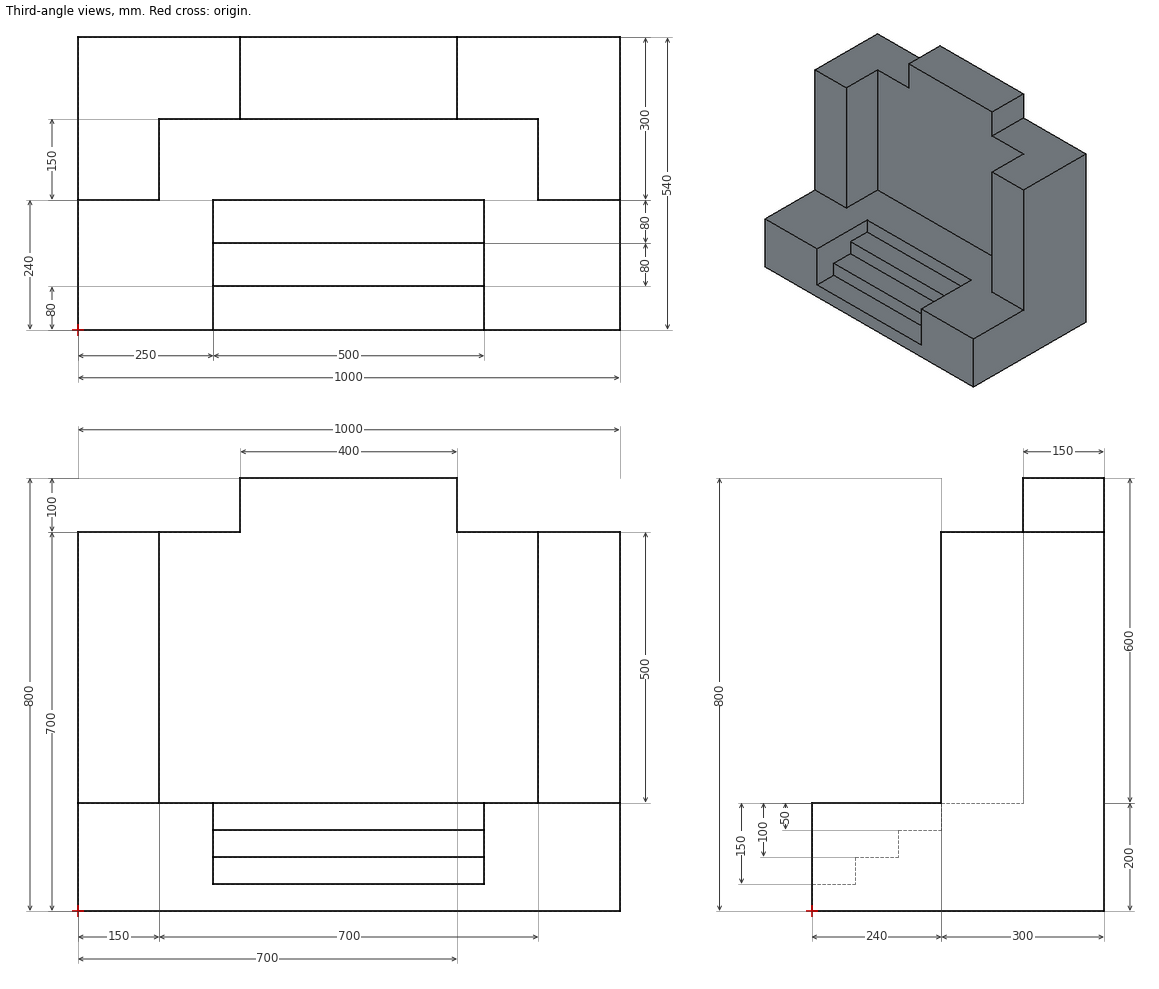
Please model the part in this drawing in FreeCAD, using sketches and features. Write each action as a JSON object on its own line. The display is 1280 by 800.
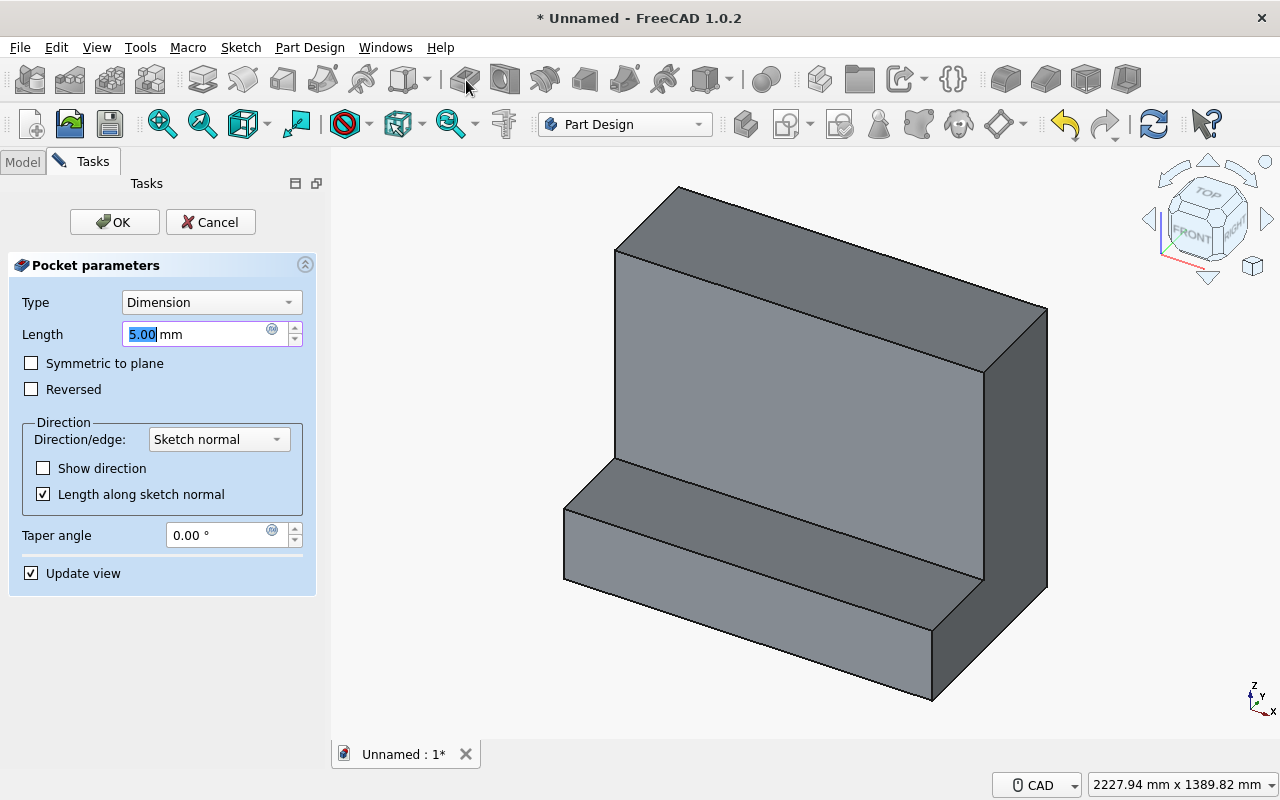
{"action": "type", "text": "100"}
{"action": "key", "text": "Tab"}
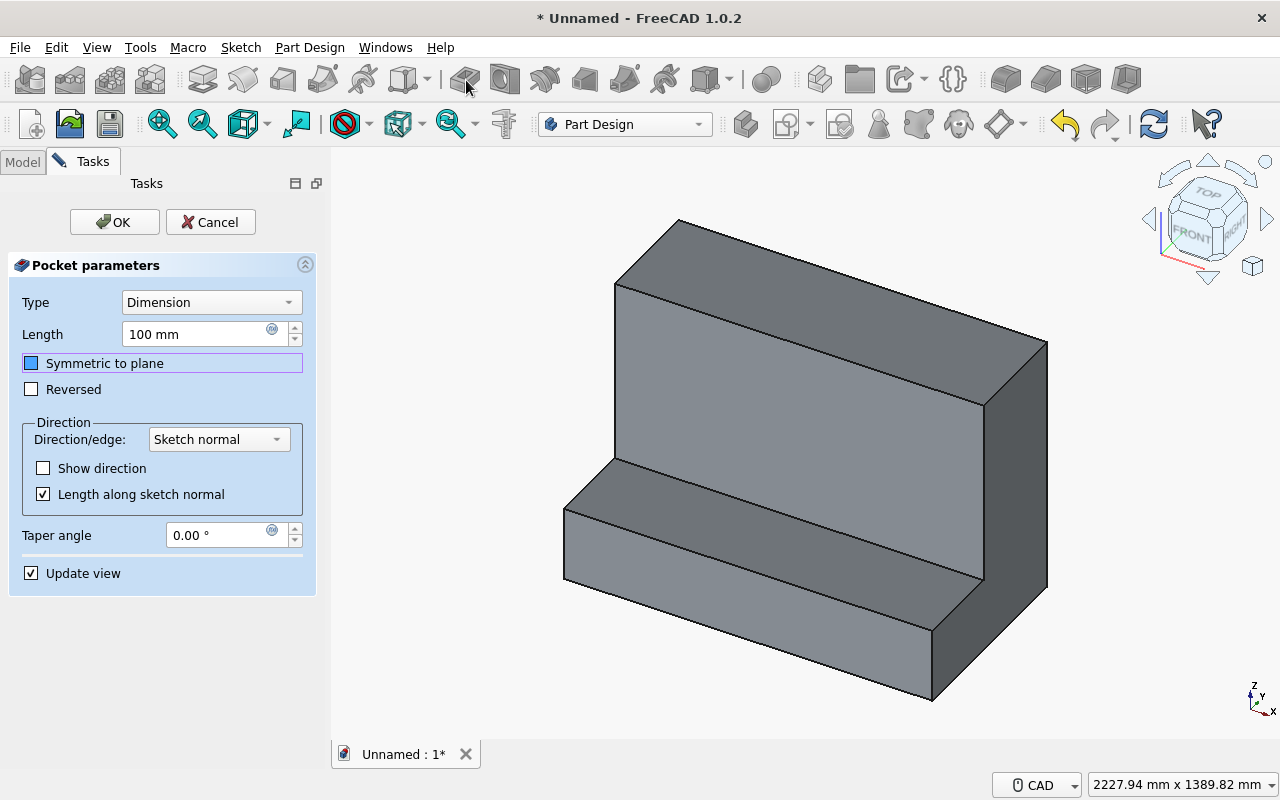
{"action": "left_click", "coordinate": [115, 222]}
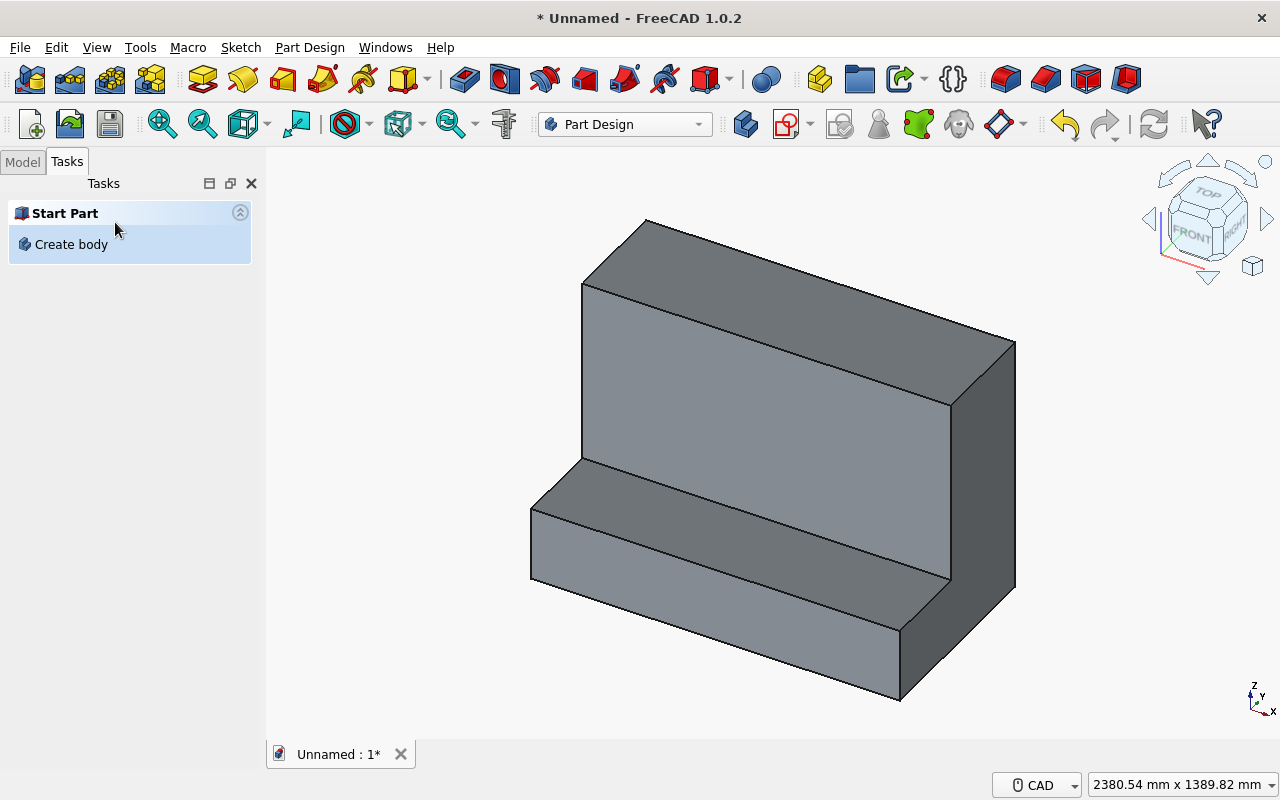
{"action": "key", "text": "4"}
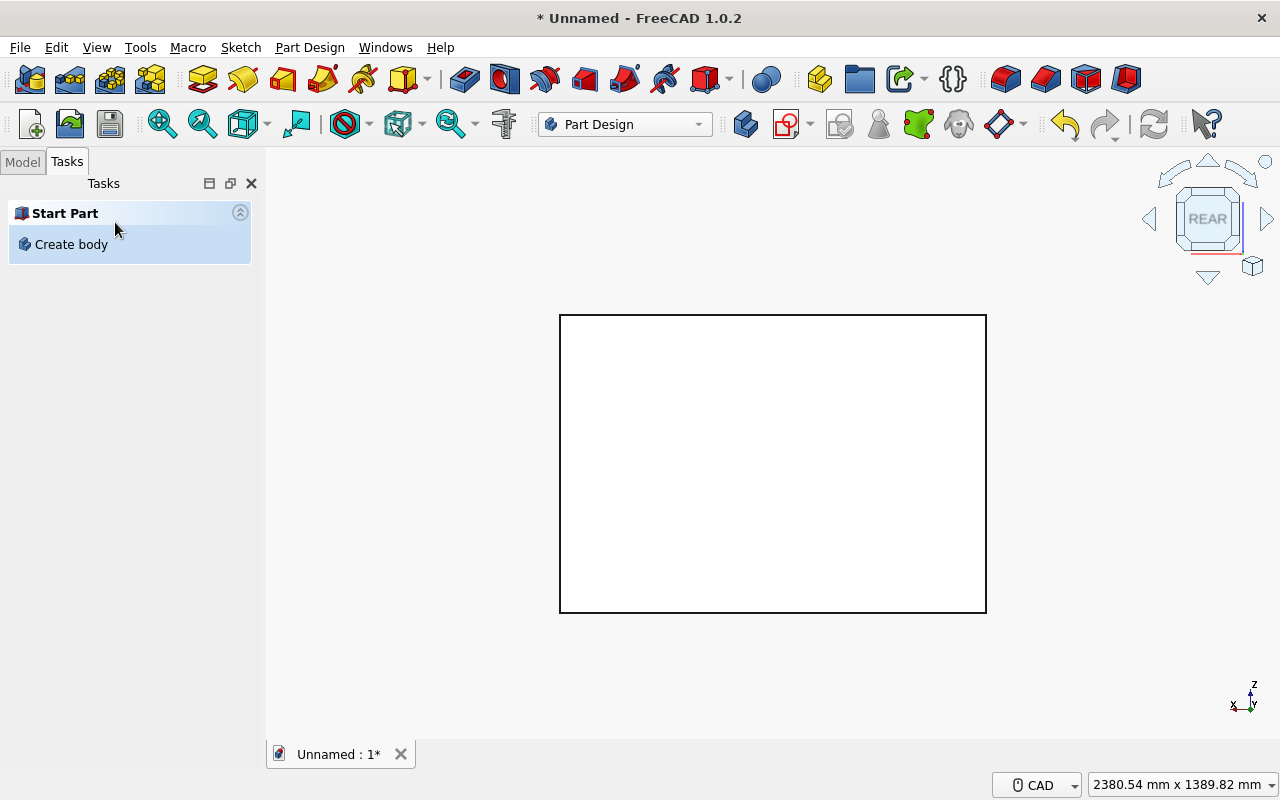
{"action": "left_click", "coordinate": [712, 463]}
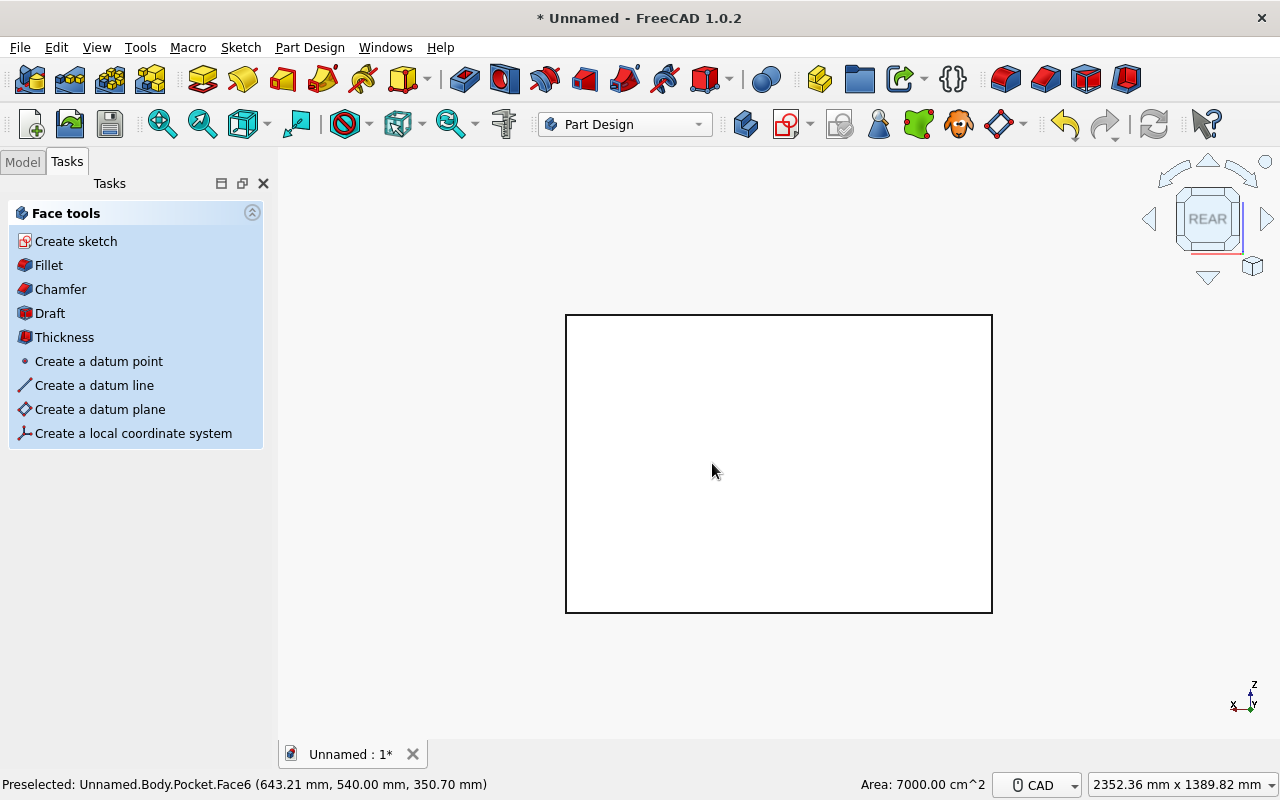
{"action": "left_click", "coordinate": [786, 124]}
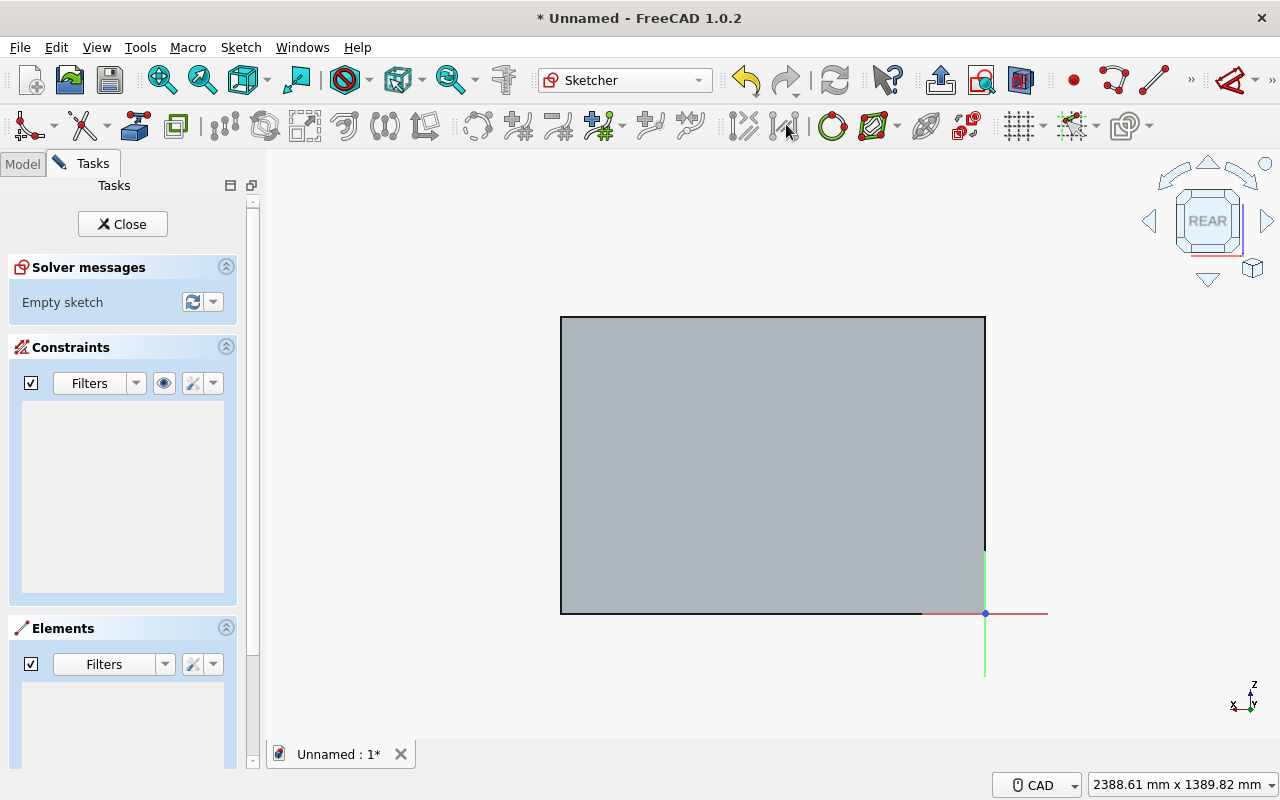
{"action": "key", "text": "g r"}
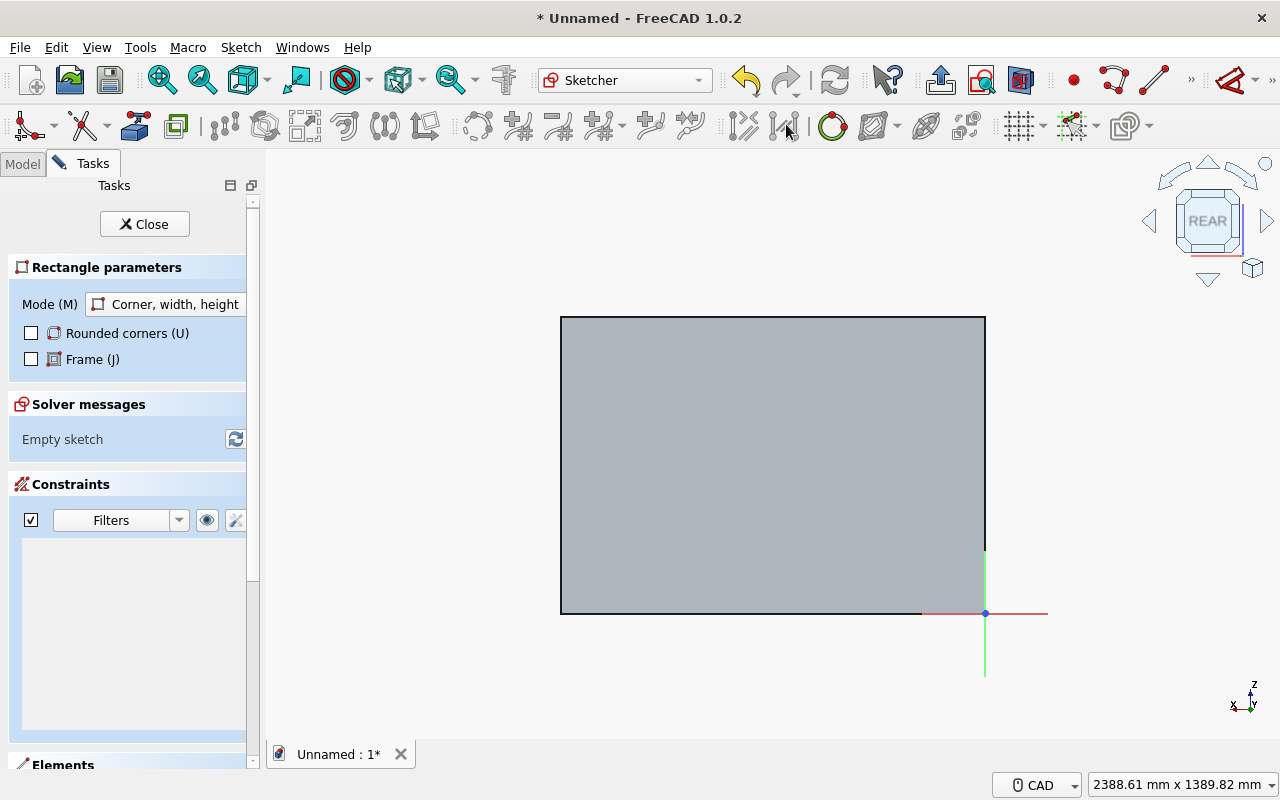
{"action": "left_click", "coordinate": [688, 274]}
{"action": "mouse_move", "coordinate": [858, 317]}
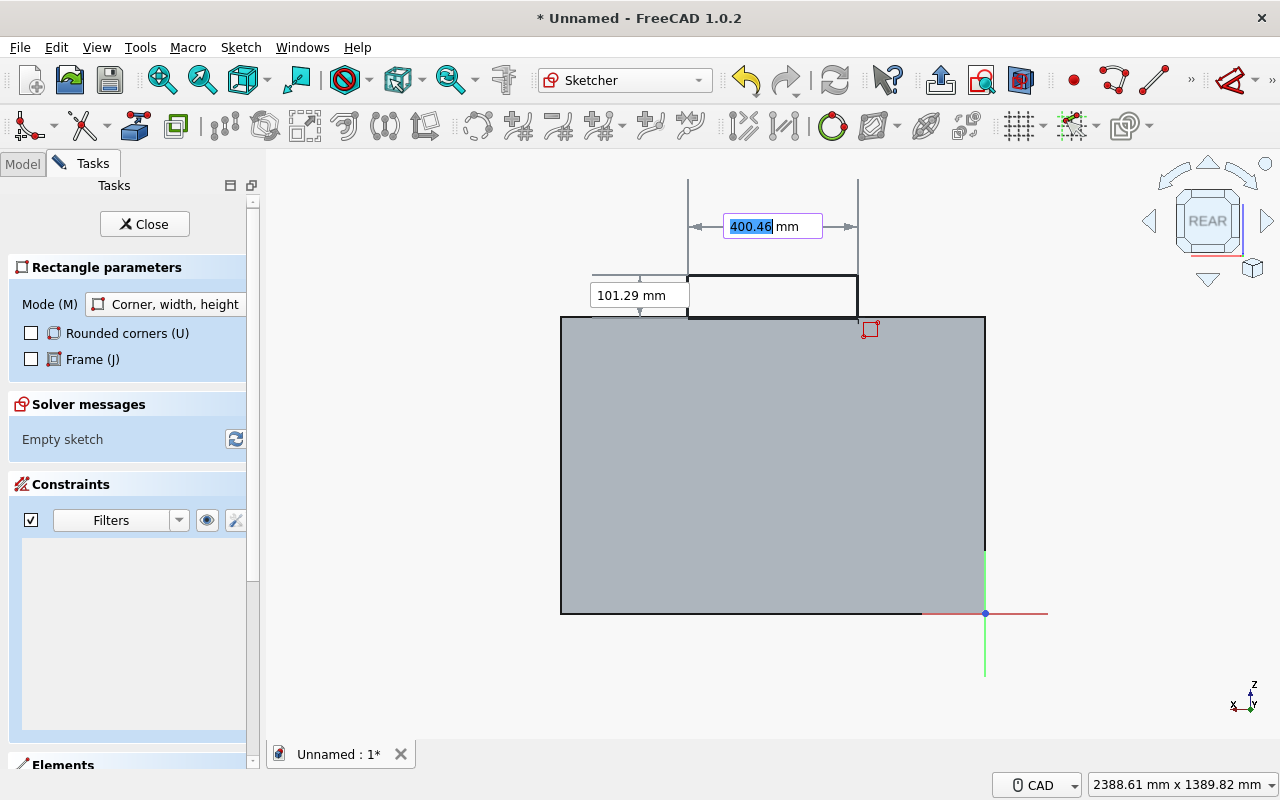
{"action": "type", "text": "400"}
{"action": "key", "text": "Tab"}
{"action": "type", "text": "100"}
{"action": "key", "text": "Return"}
{"action": "key", "text": "Escape"}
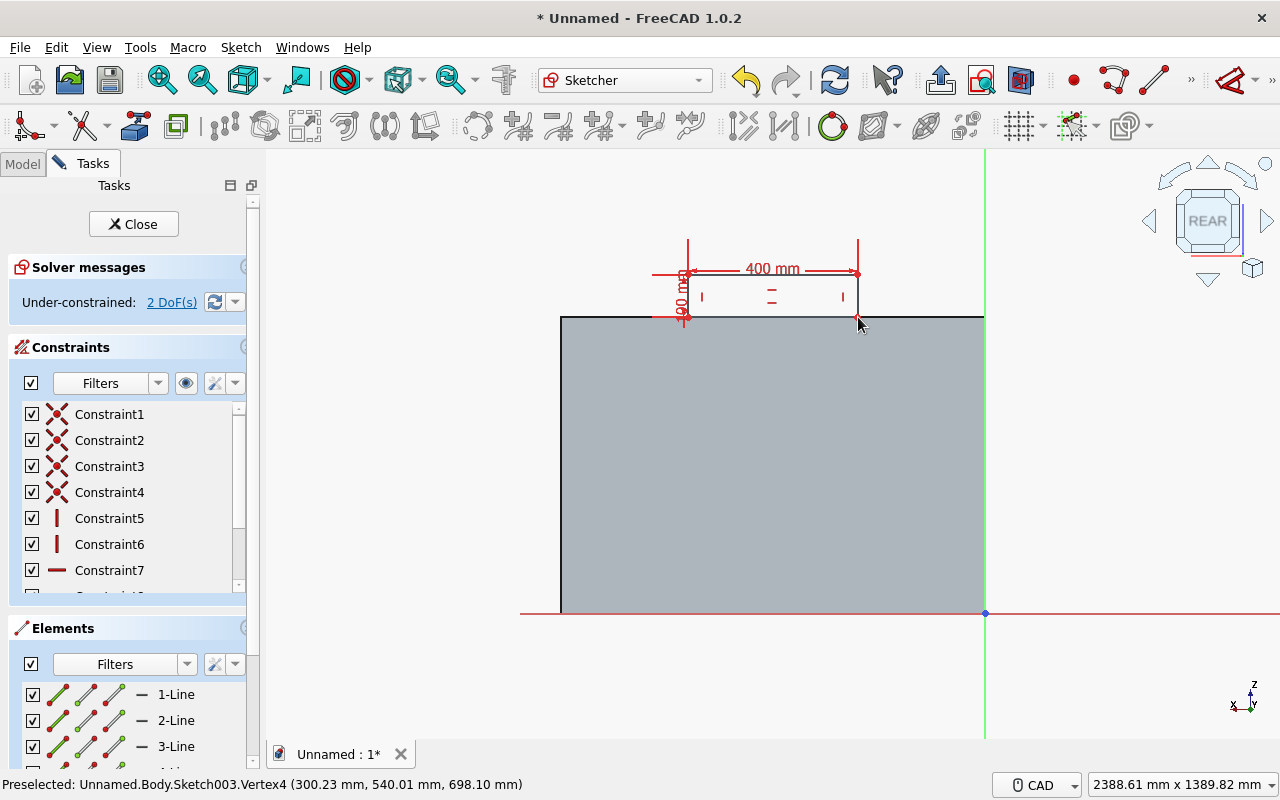
{"action": "left_click", "coordinate": [1230, 80]}